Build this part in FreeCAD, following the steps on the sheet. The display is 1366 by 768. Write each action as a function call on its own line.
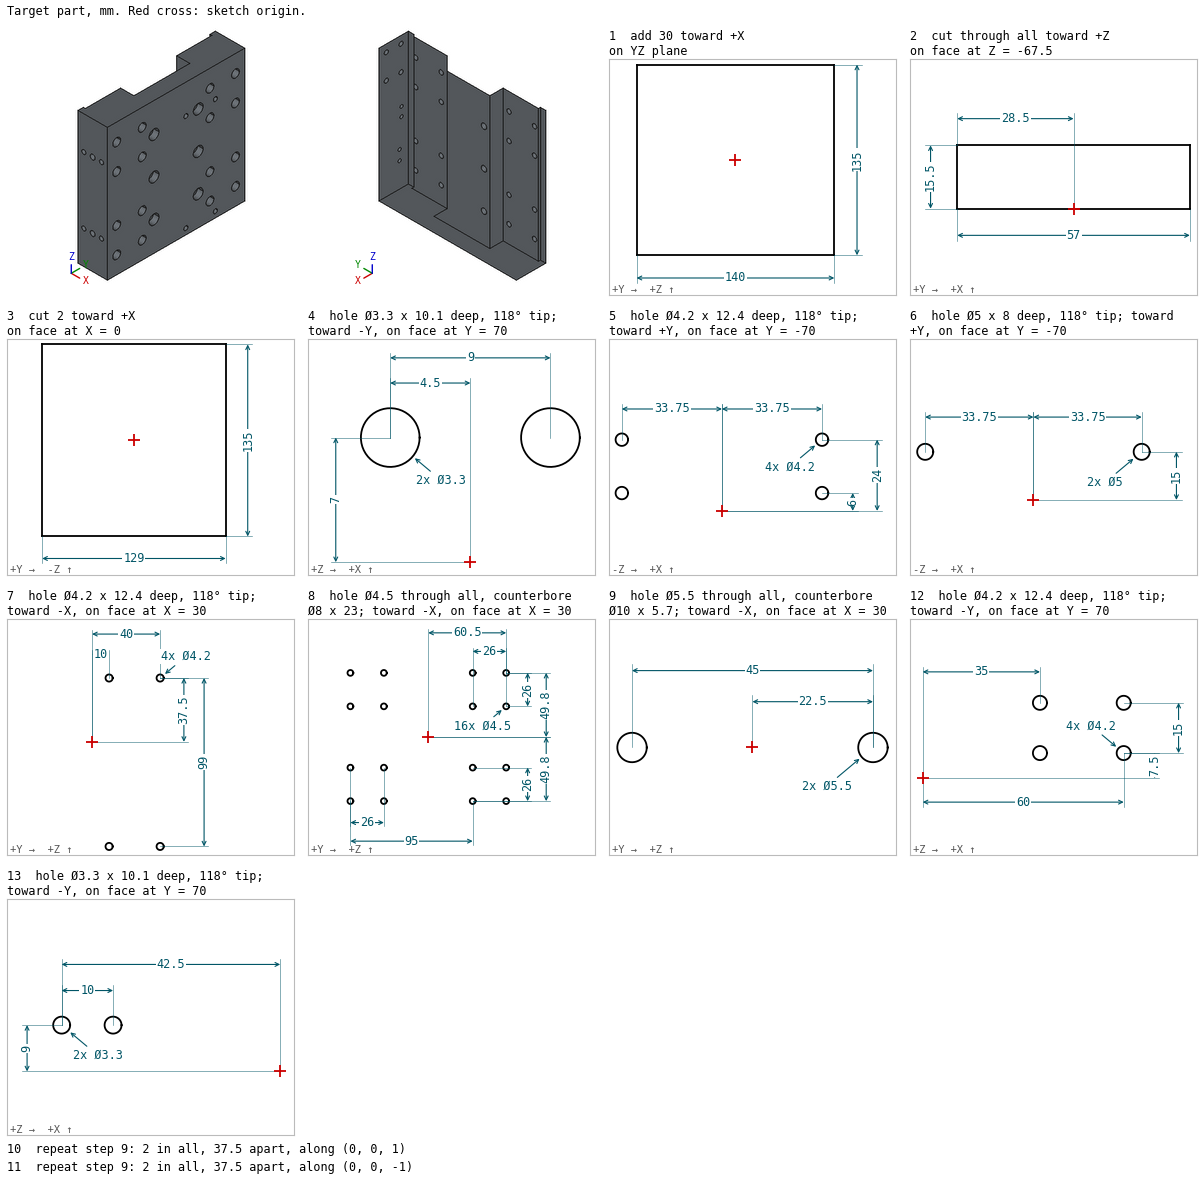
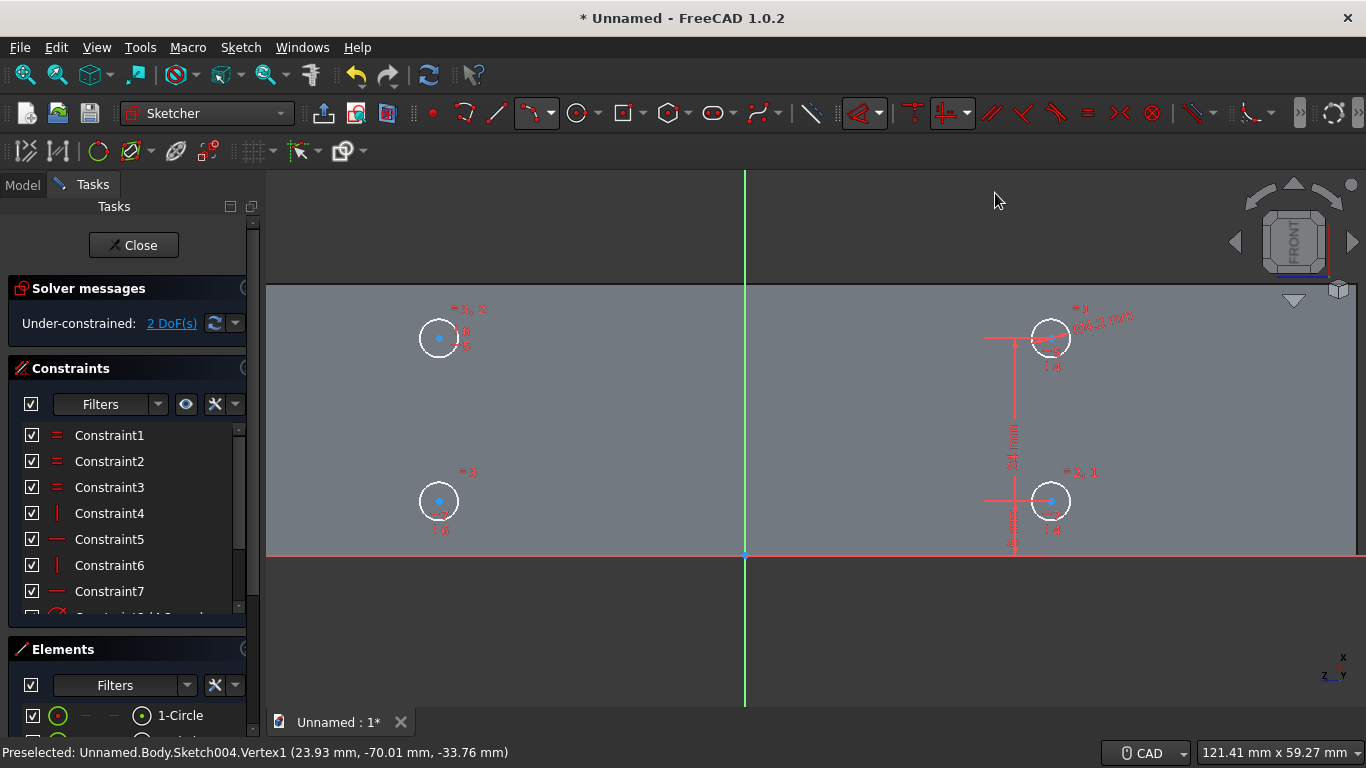
click(1051, 338)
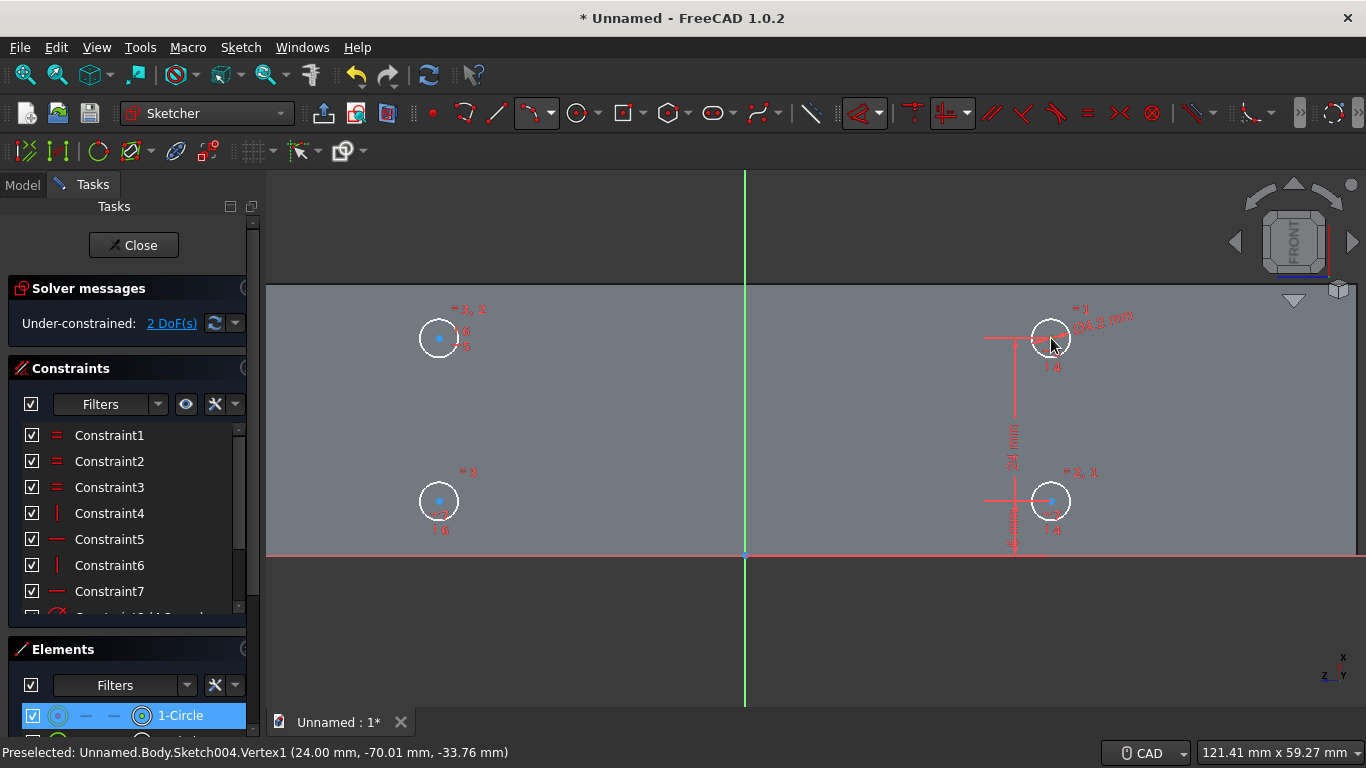
key(l)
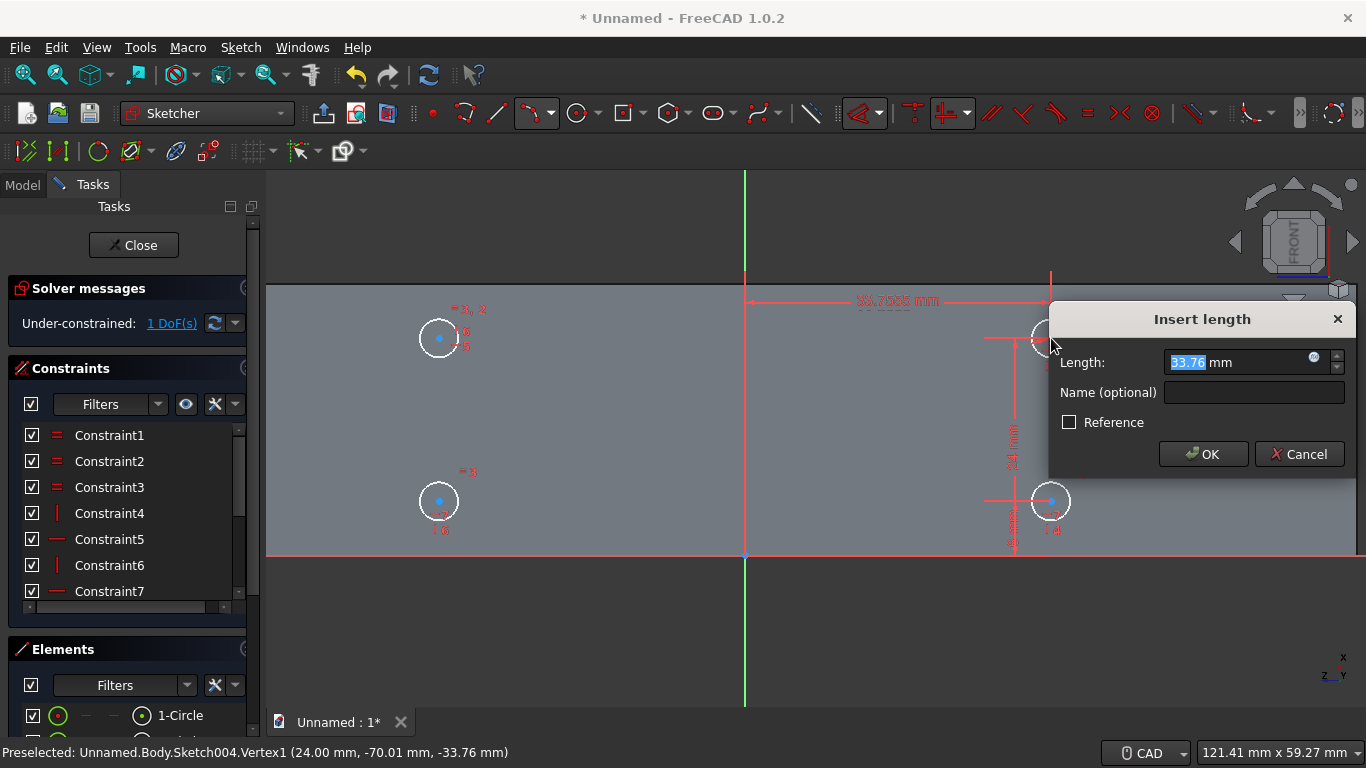
text(33.75)
key(Return)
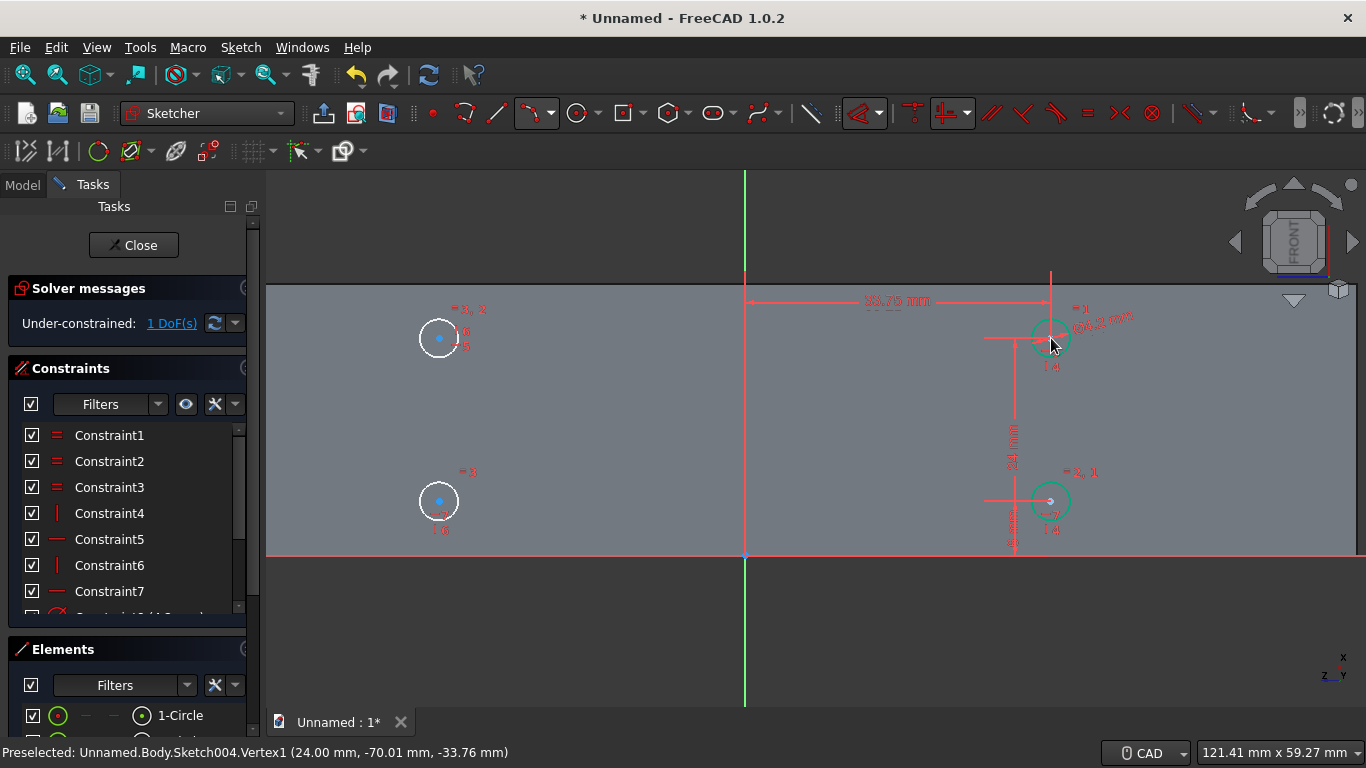
click(439, 338)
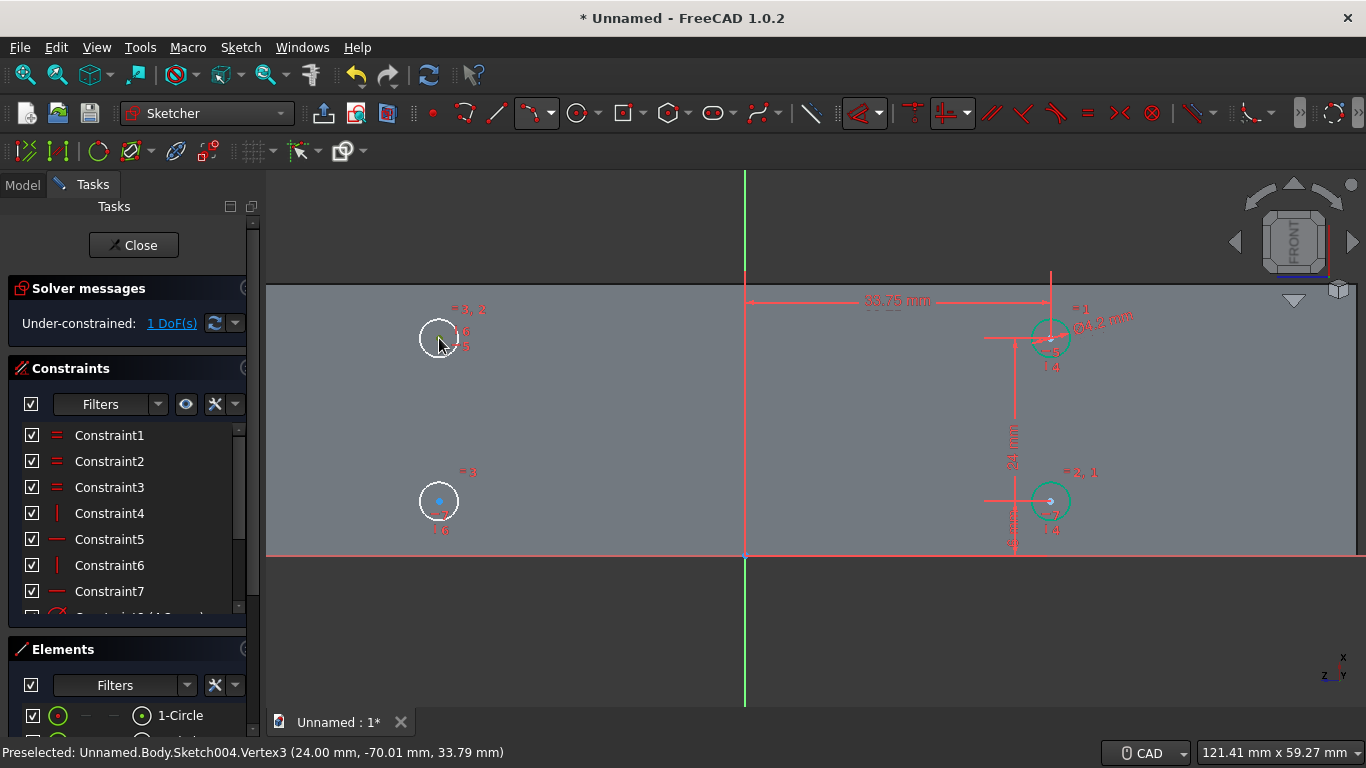
click(882, 114)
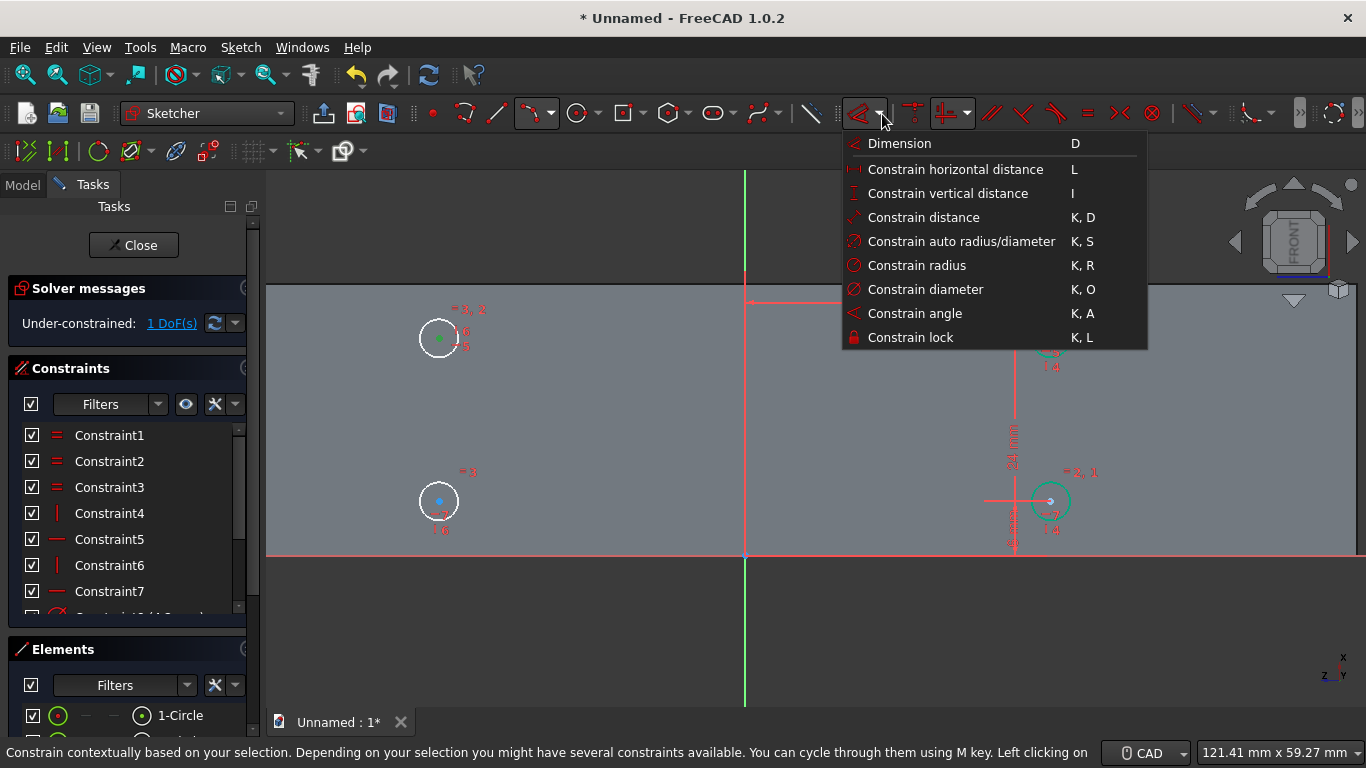
click(995, 169)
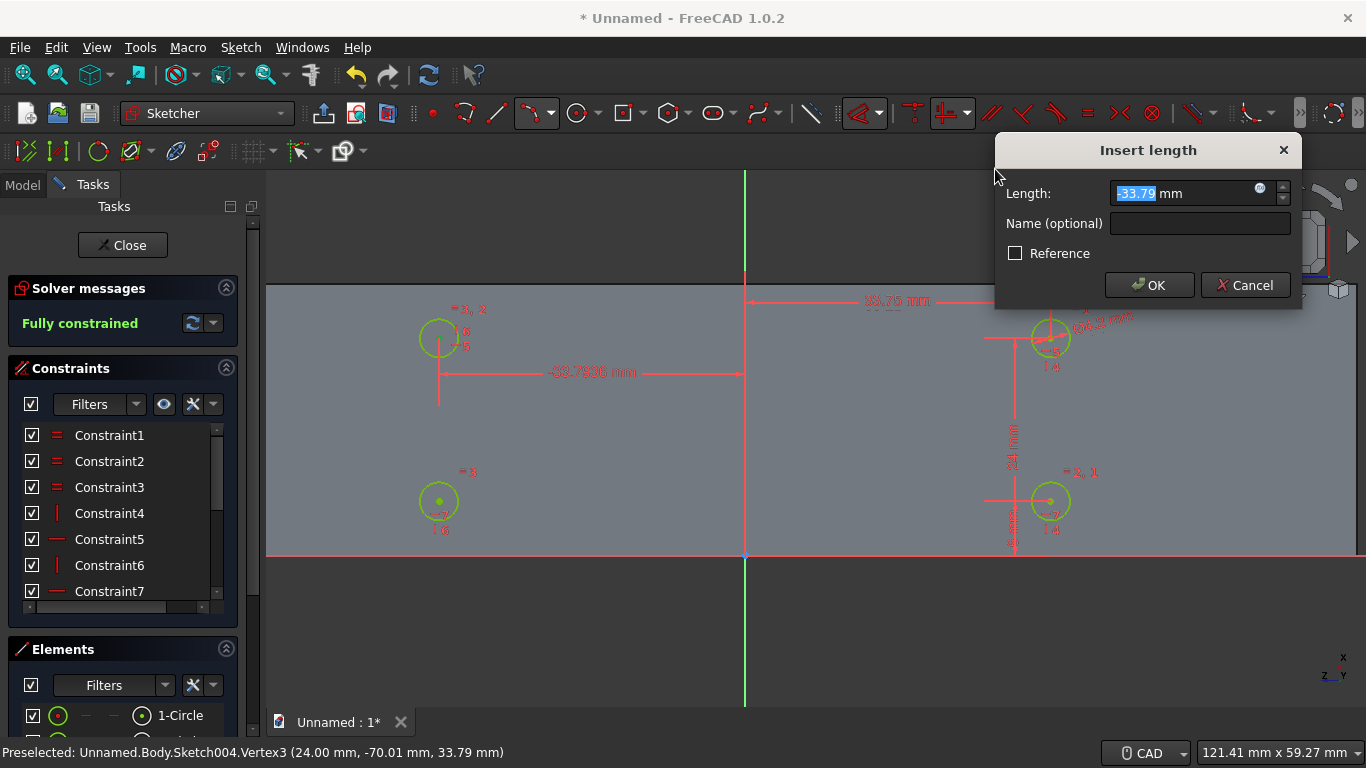
text(-33.75)
key(Return)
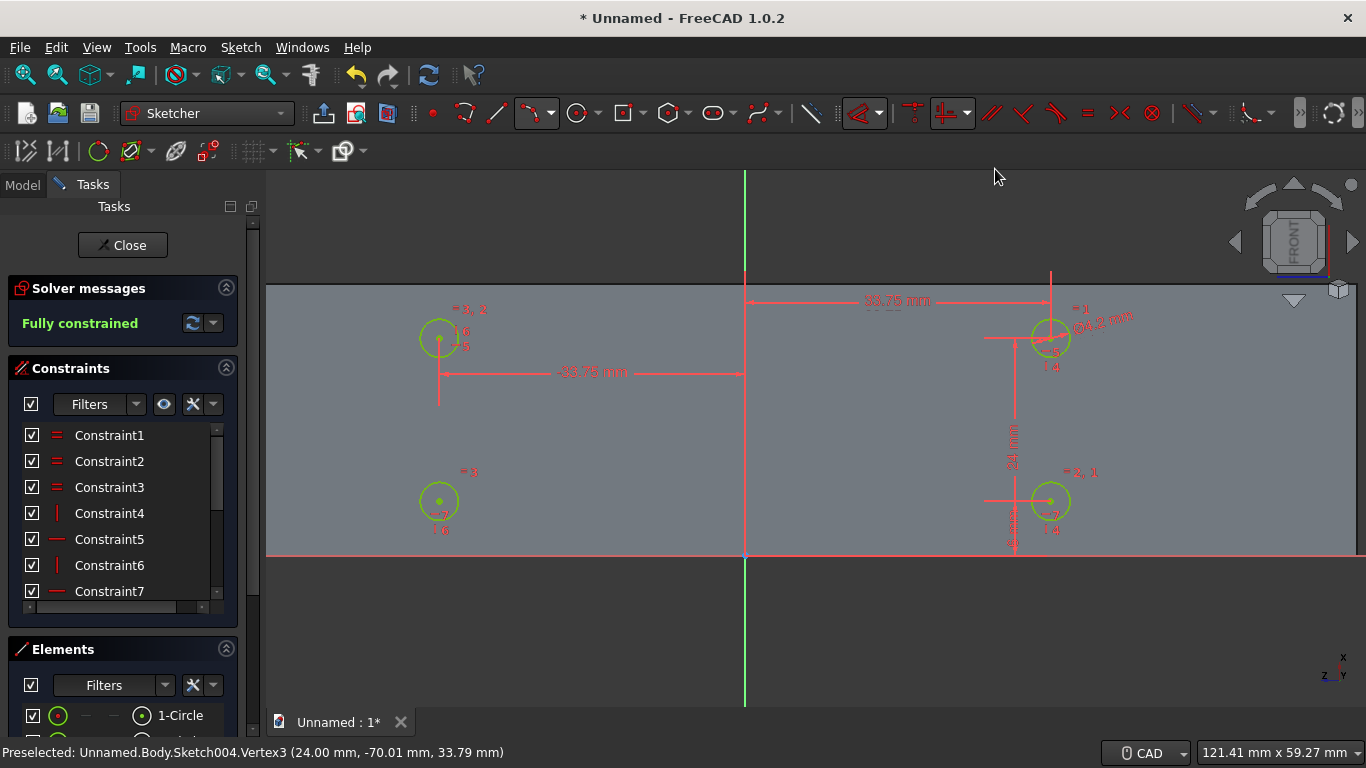
click(123, 245)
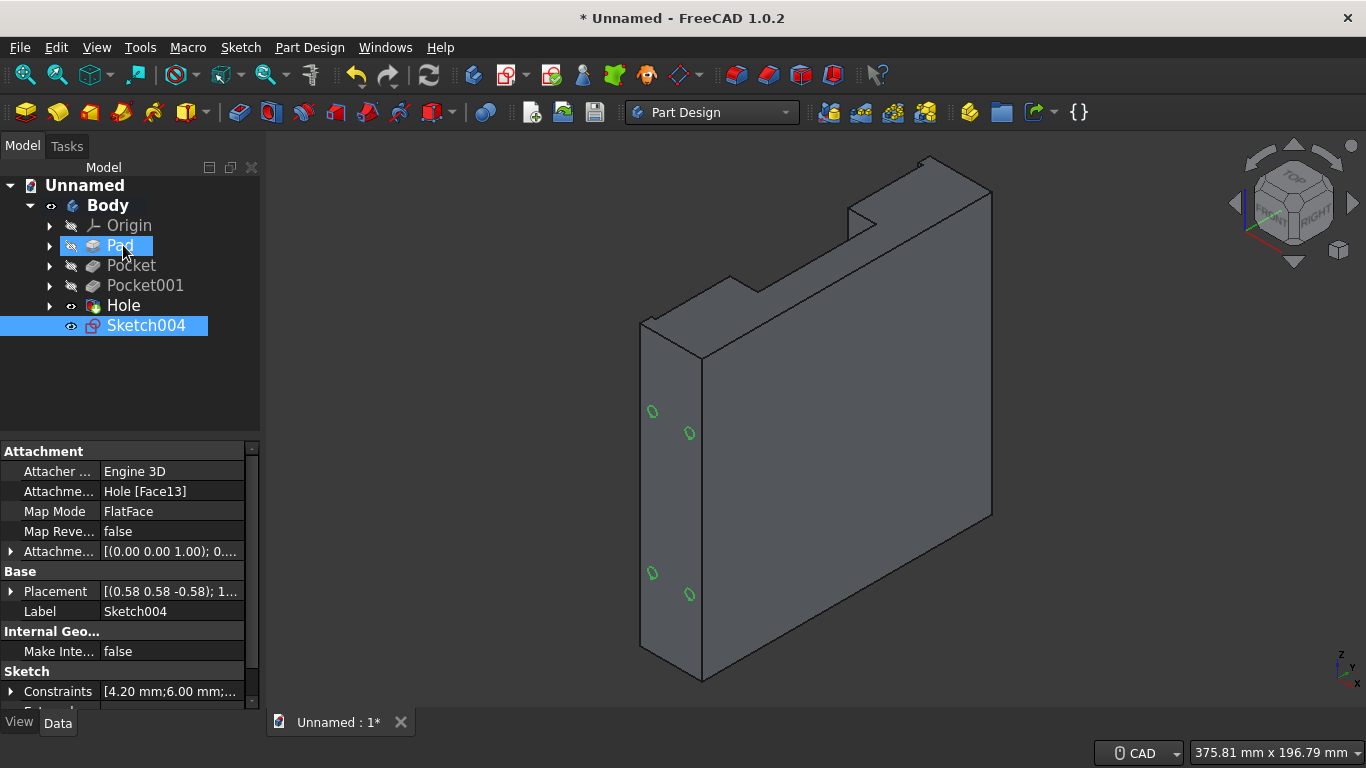
click(272, 112)